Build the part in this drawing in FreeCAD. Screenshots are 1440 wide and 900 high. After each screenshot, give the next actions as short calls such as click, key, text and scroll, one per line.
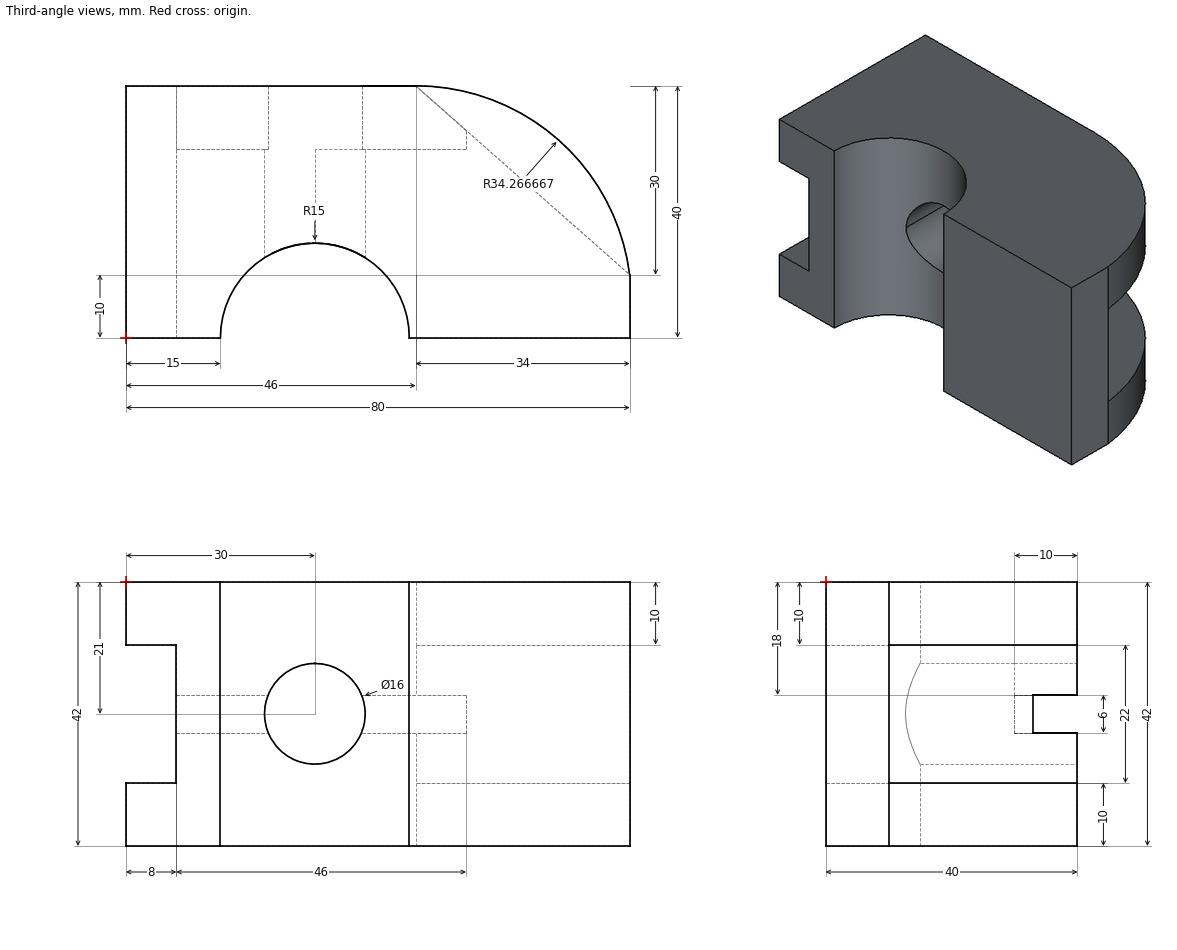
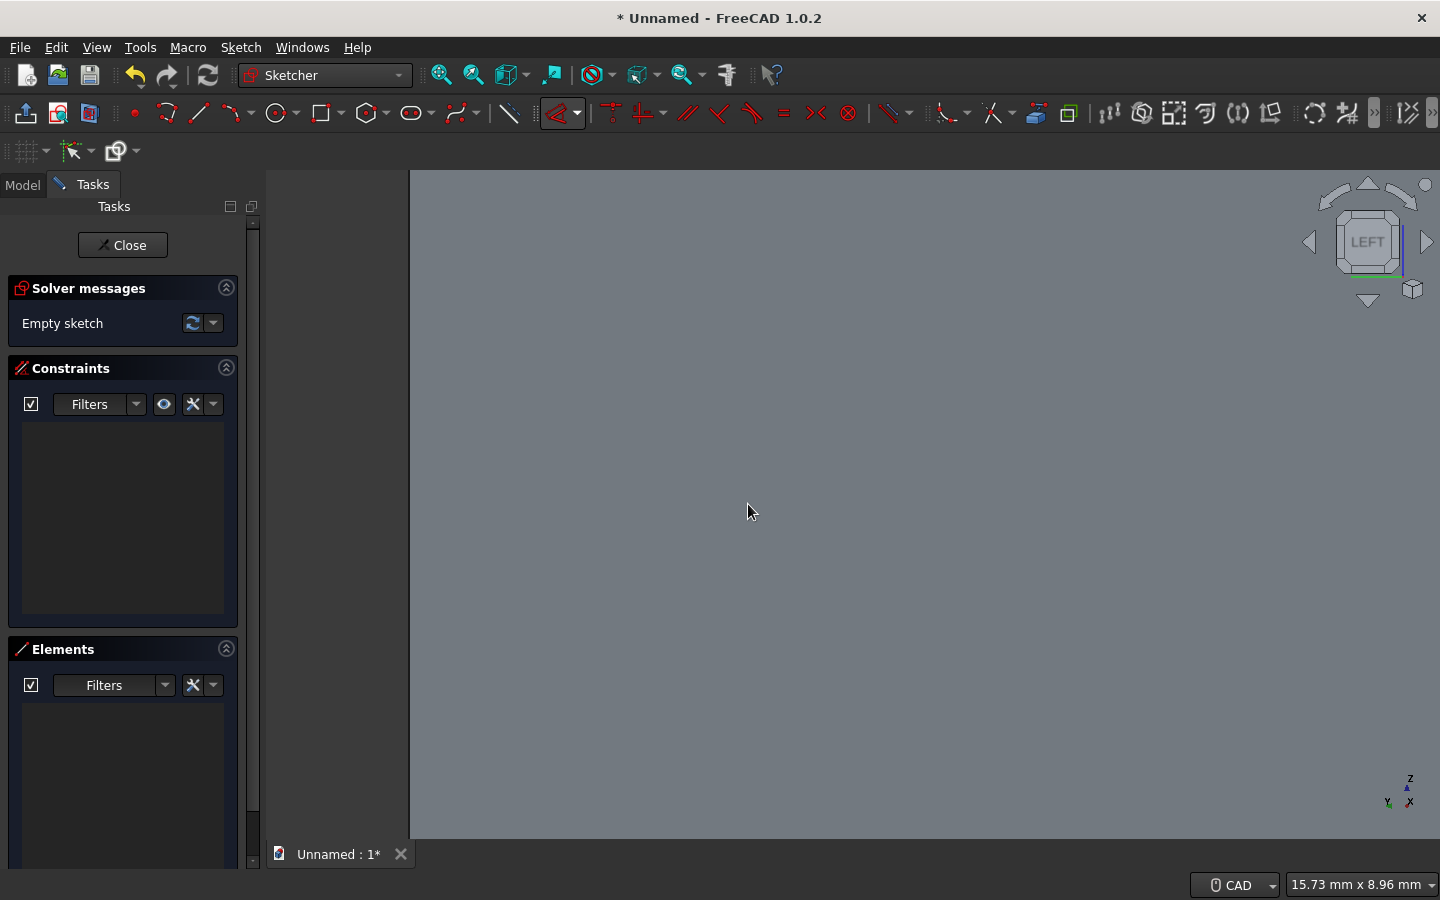
click(322, 114)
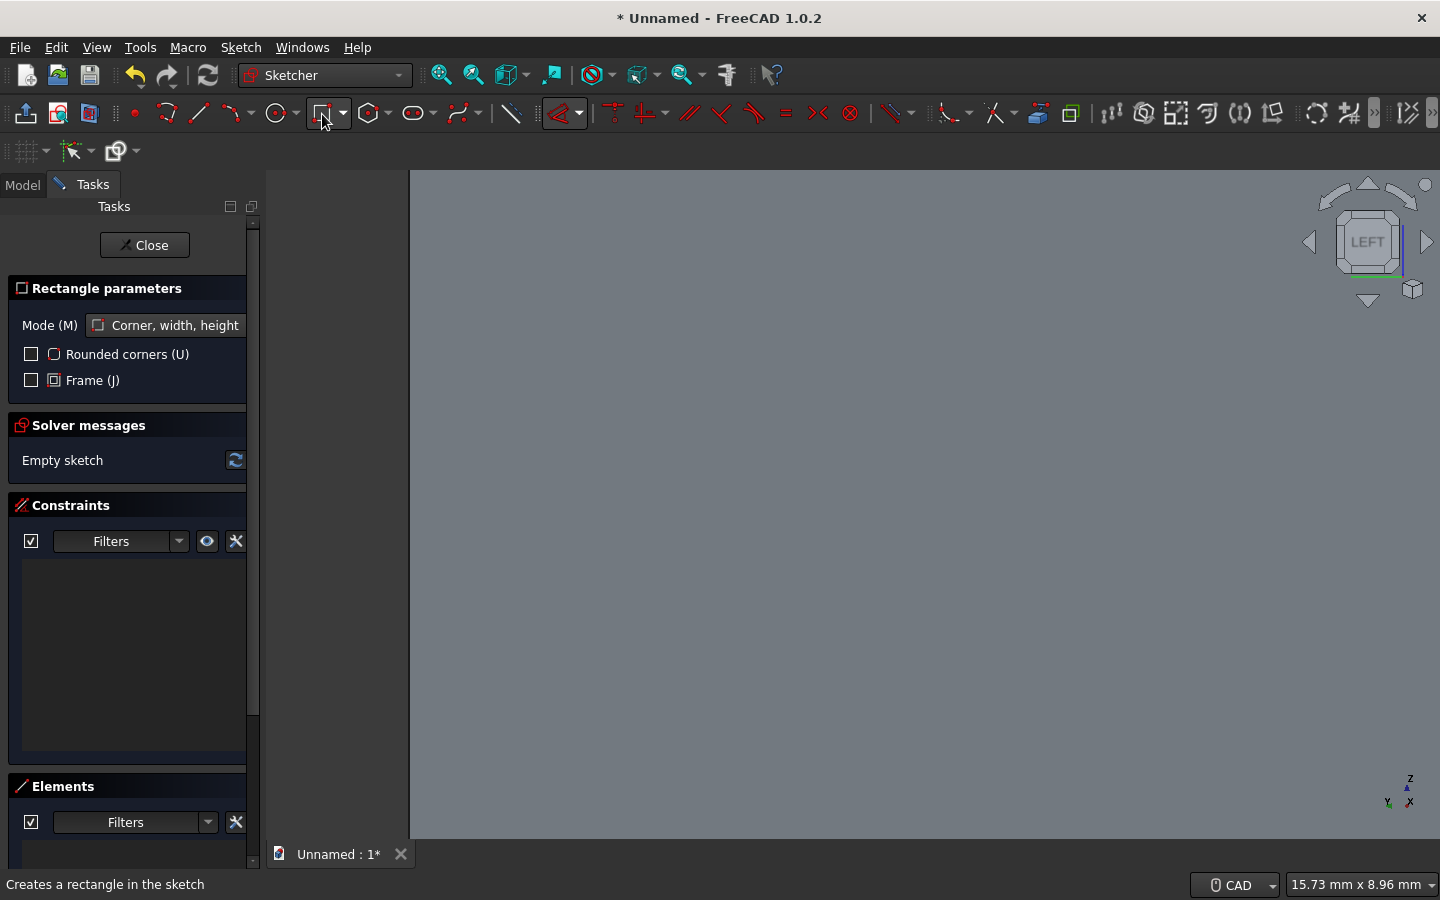
click(409, 281)
move(1155, 728)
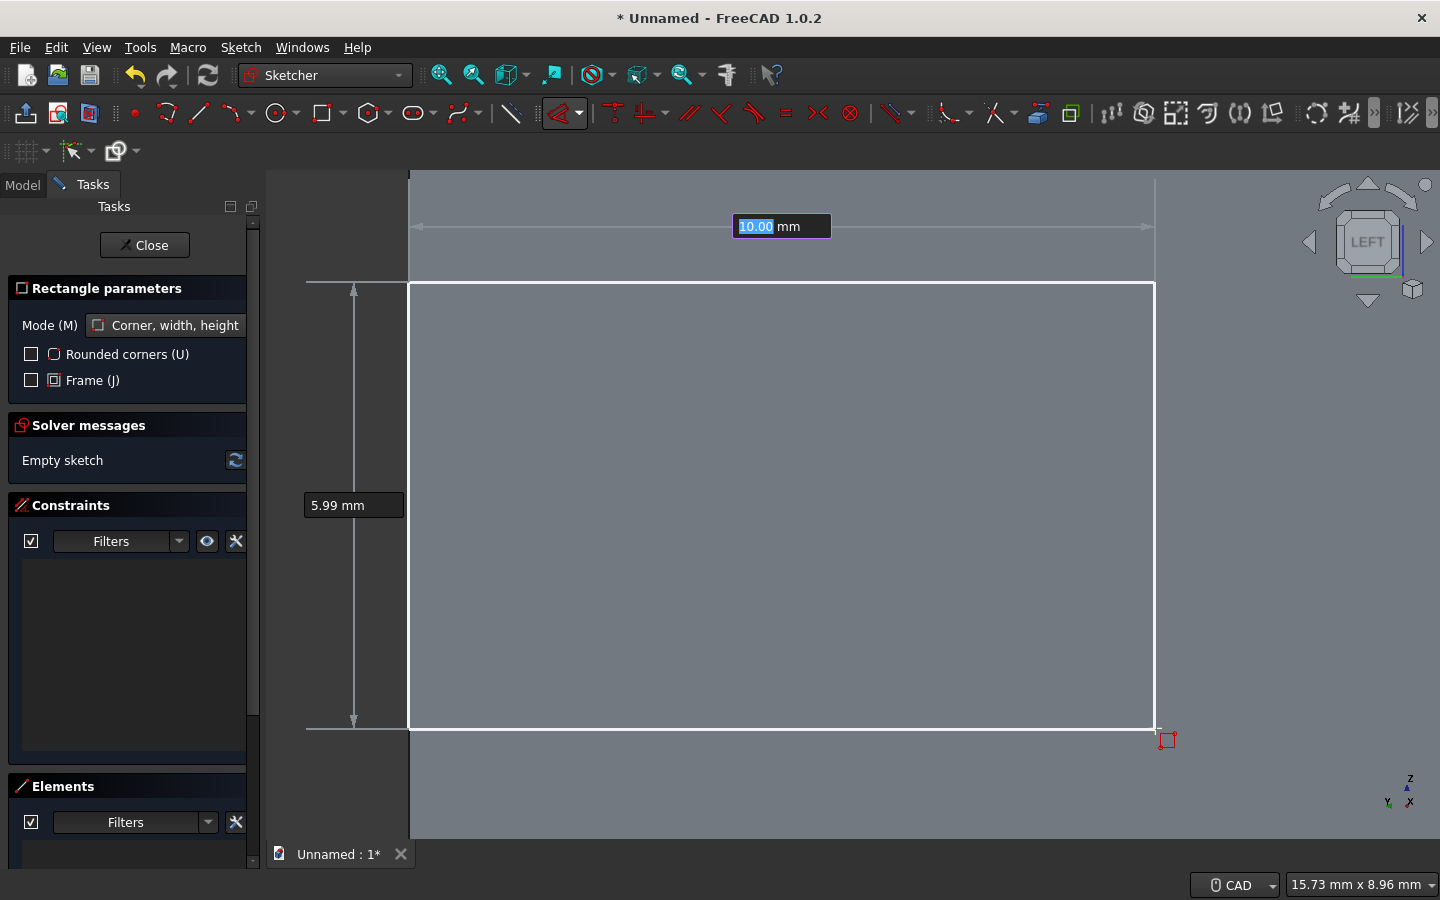
text(10)
key(Tab)
text(6)
key(Return)
key(Escape)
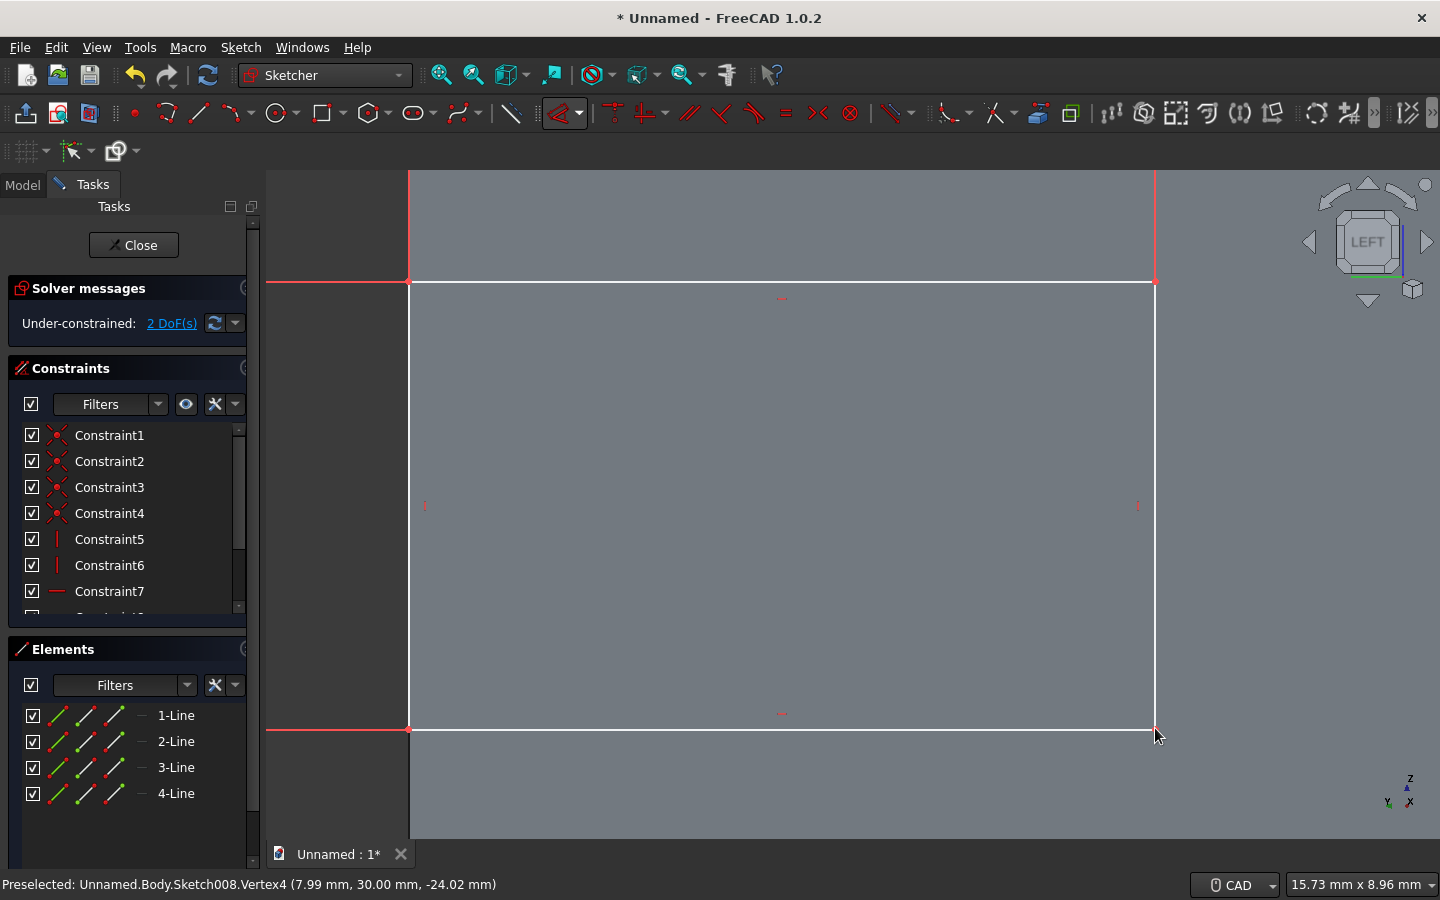
click(409, 282)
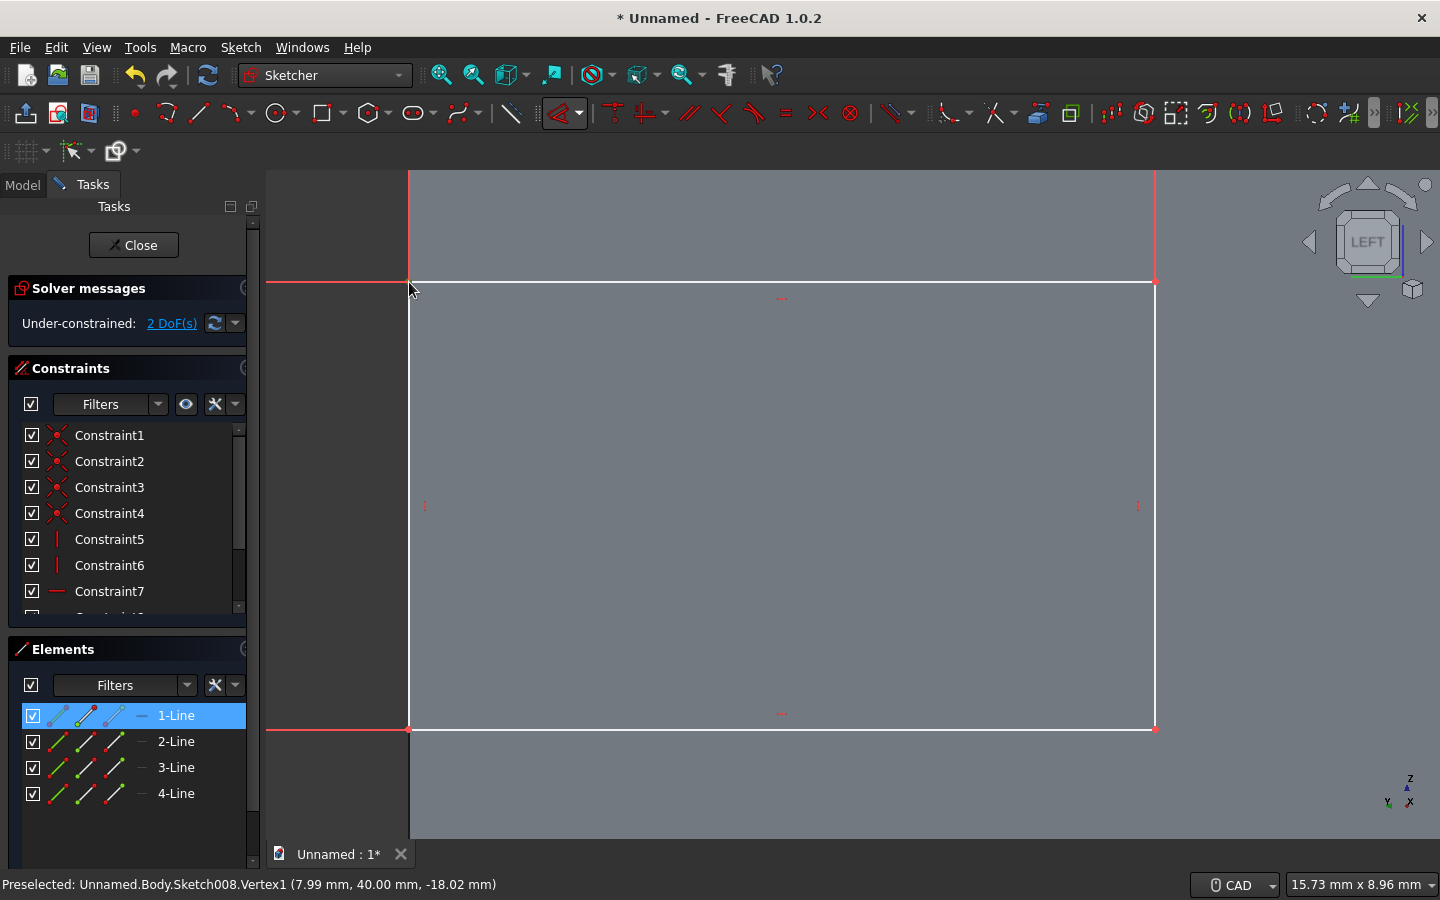
click(582, 114)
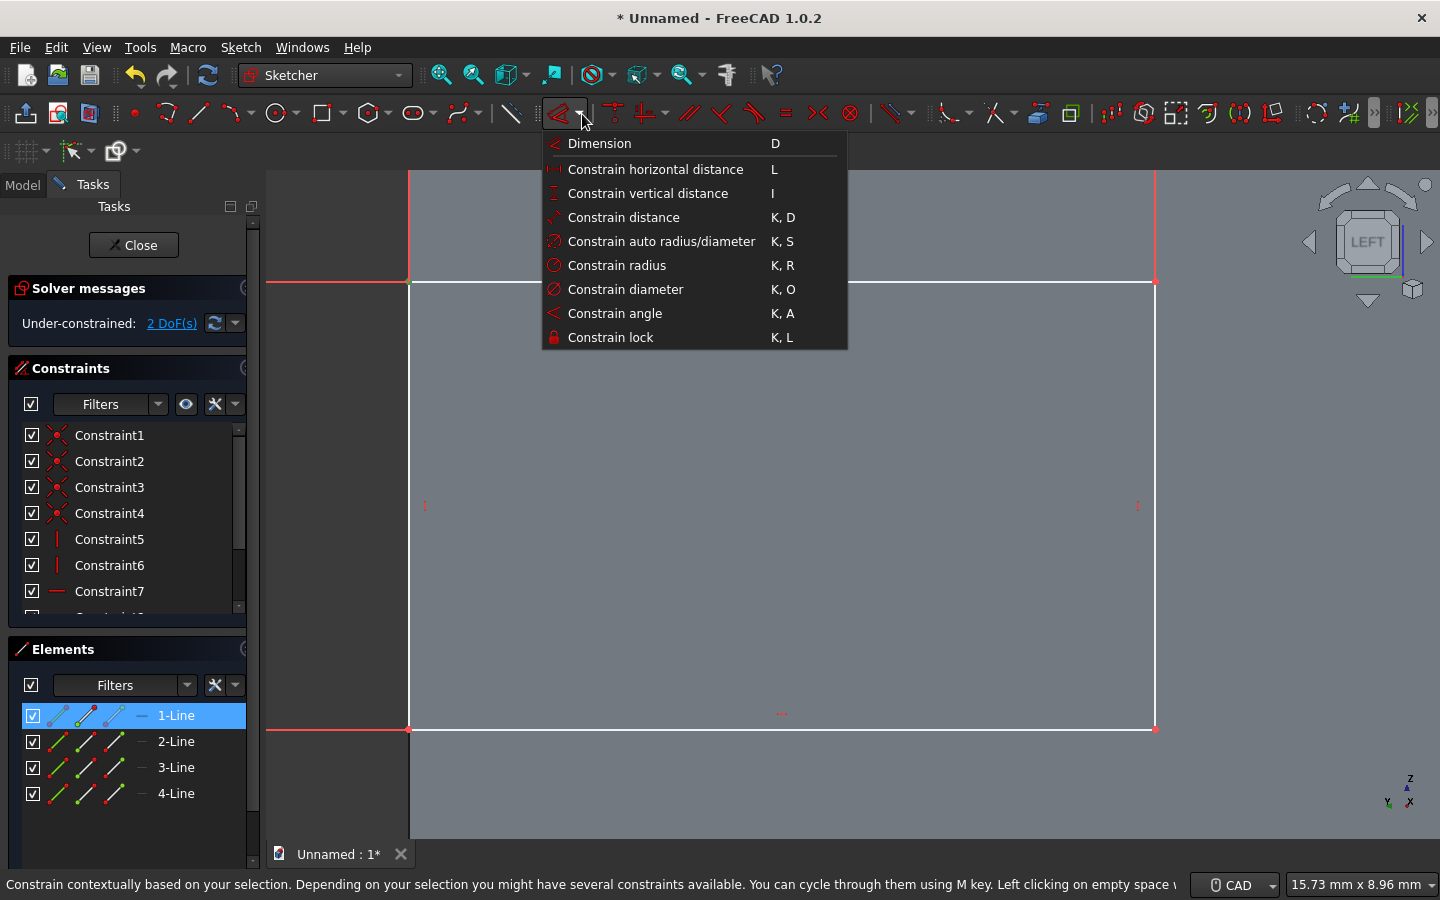
click(695, 169)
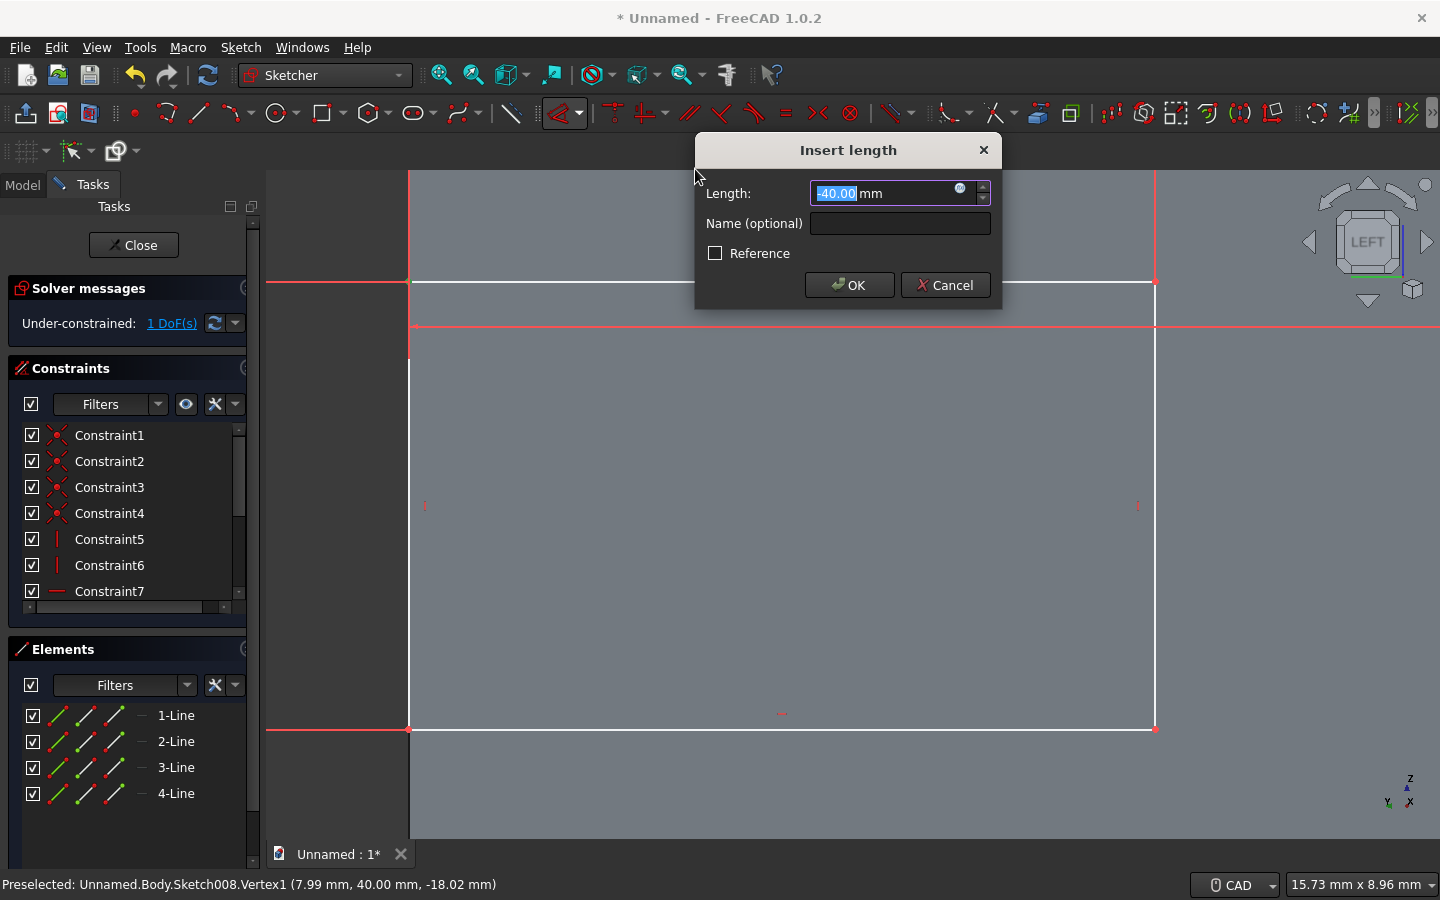
text(-40)
key(Return)